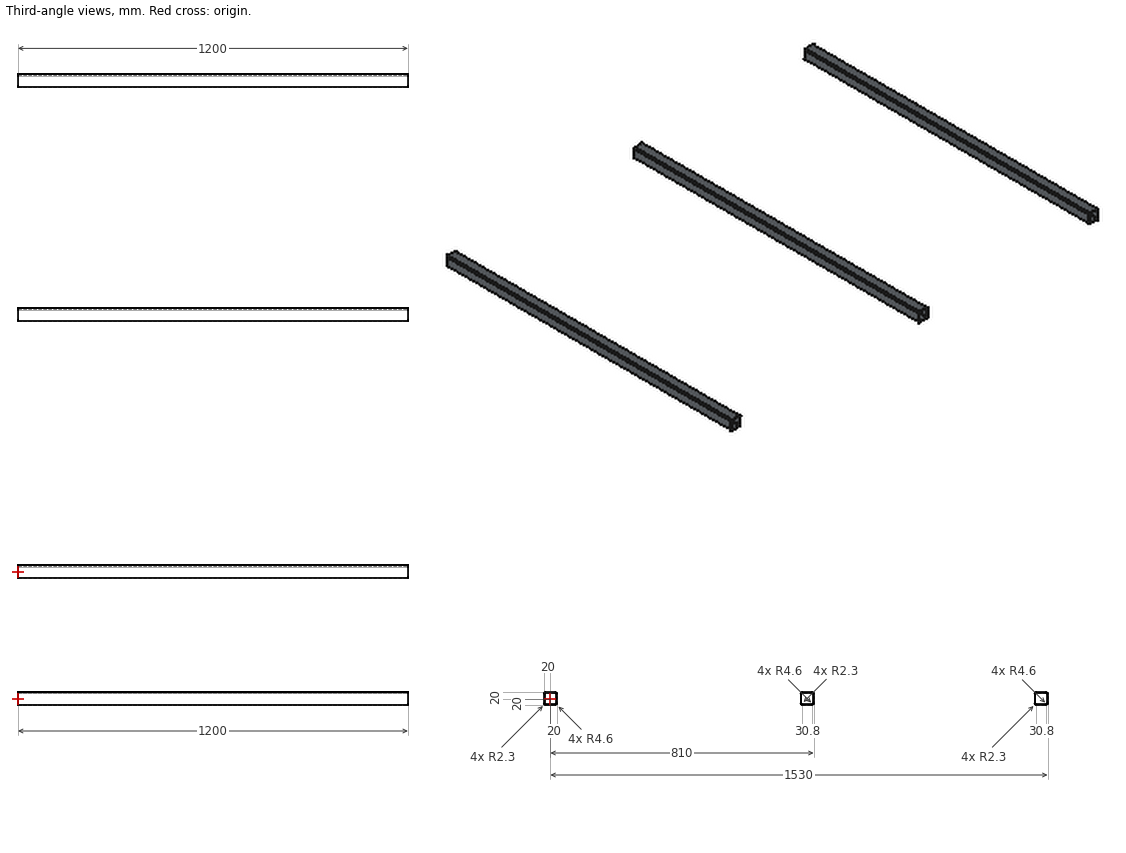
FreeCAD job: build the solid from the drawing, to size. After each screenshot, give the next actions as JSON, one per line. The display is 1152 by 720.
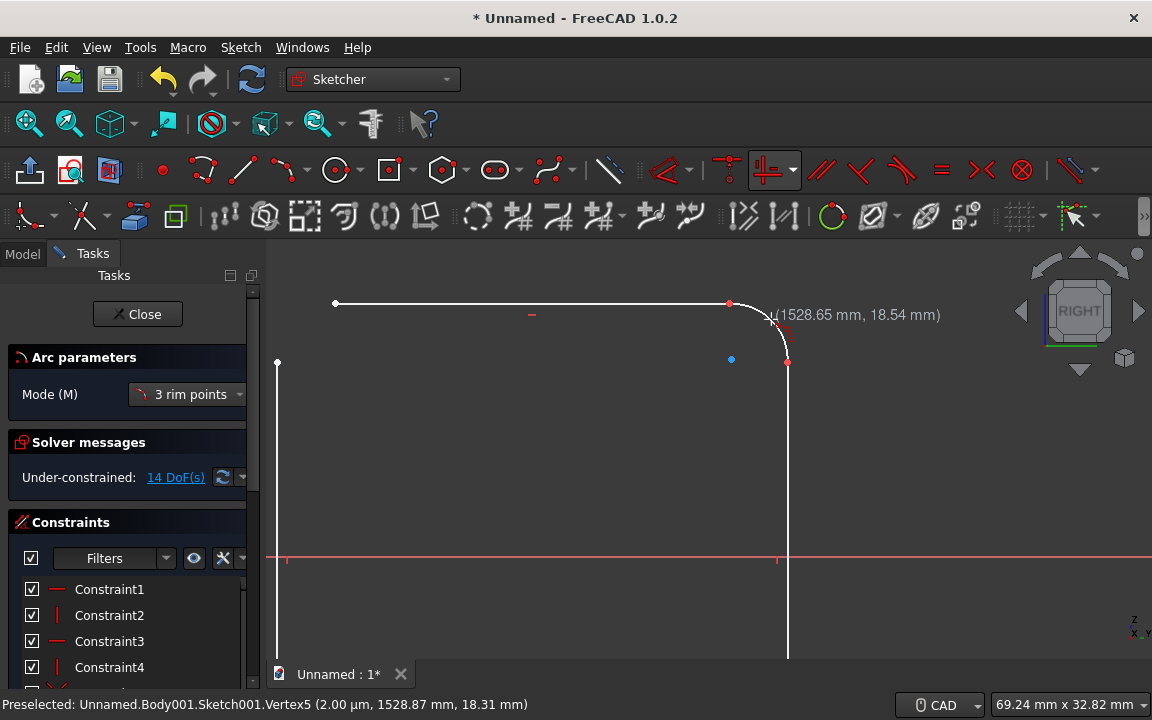
{"action": "left_click", "coordinate": [336, 304]}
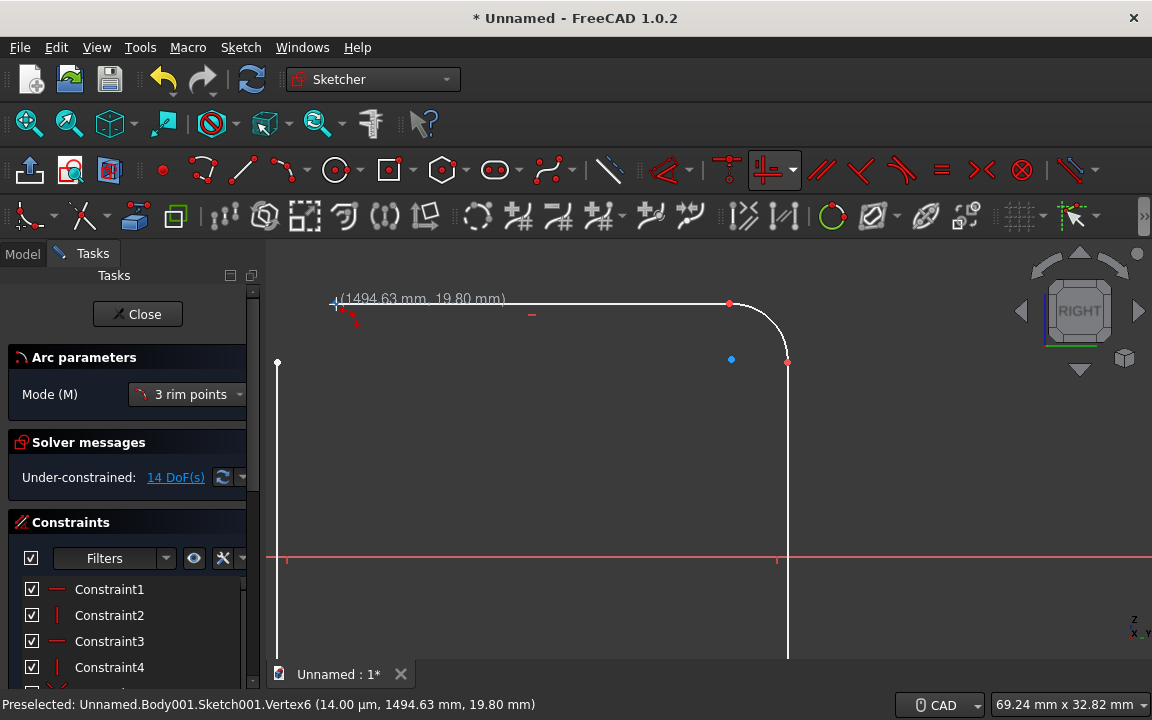
{"action": "scroll", "coordinate": [772, 317], "scroll_direction": "down", "scroll_amount": 3}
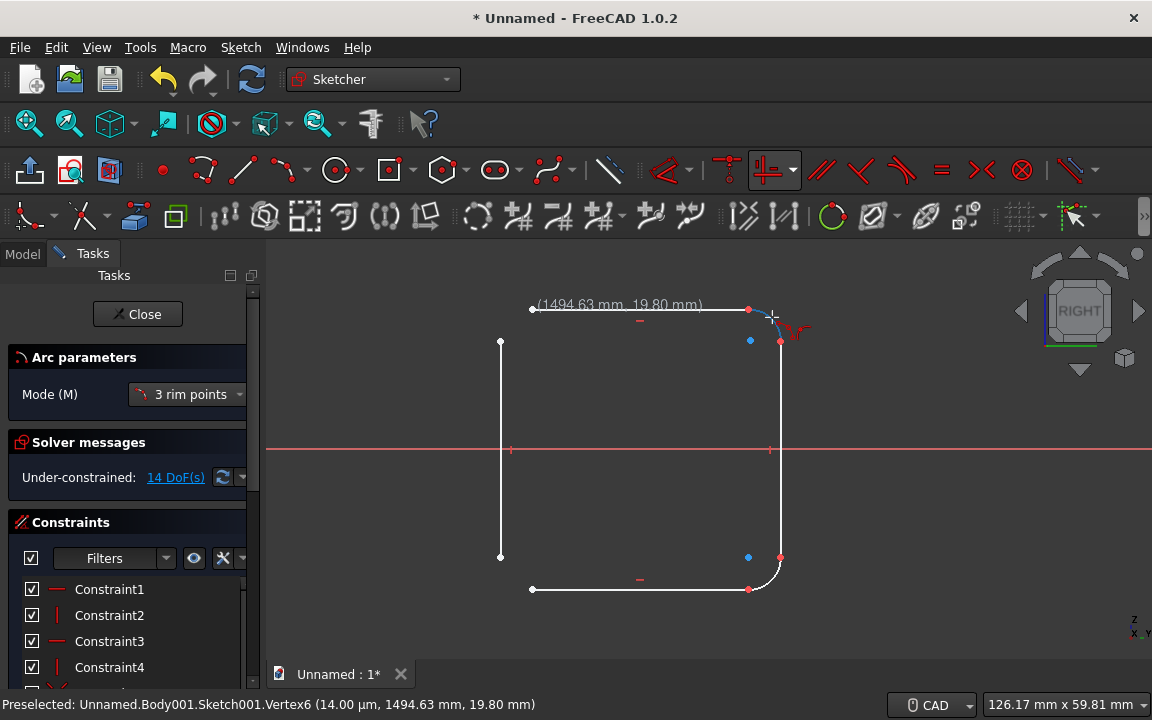
{"action": "left_click", "coordinate": [501, 342]}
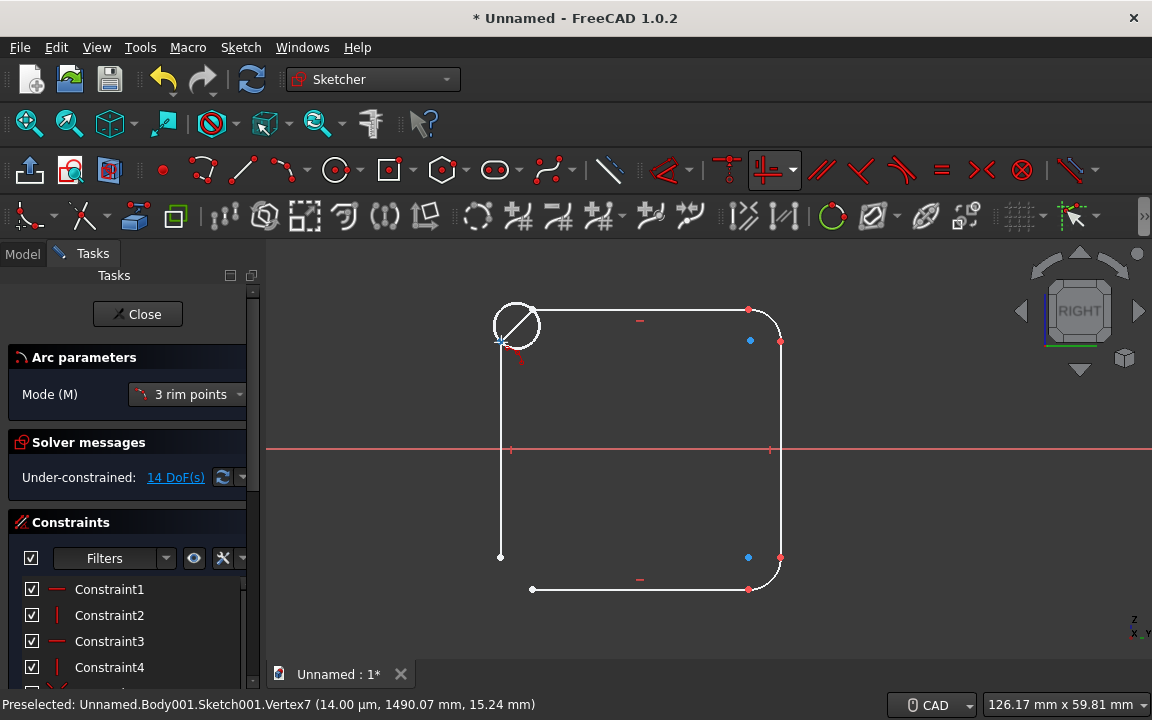
{"action": "scroll", "coordinate": [510, 318], "scroll_direction": "up", "scroll_amount": 3}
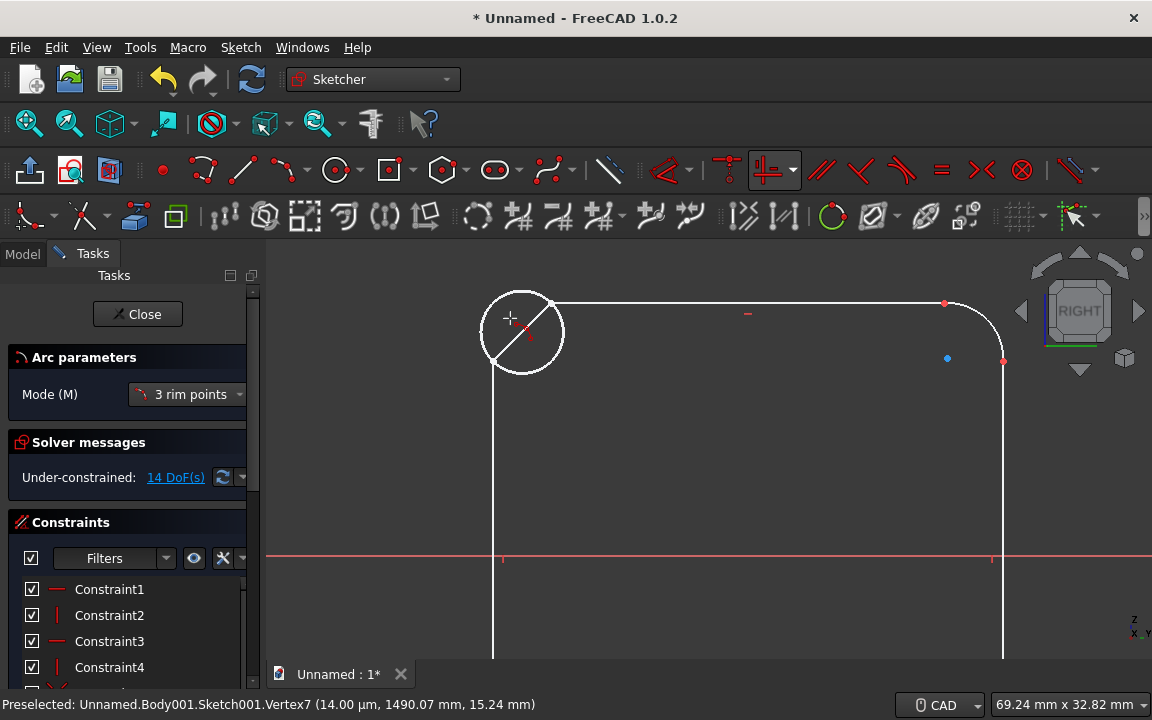
{"action": "left_click", "coordinate": [509, 318]}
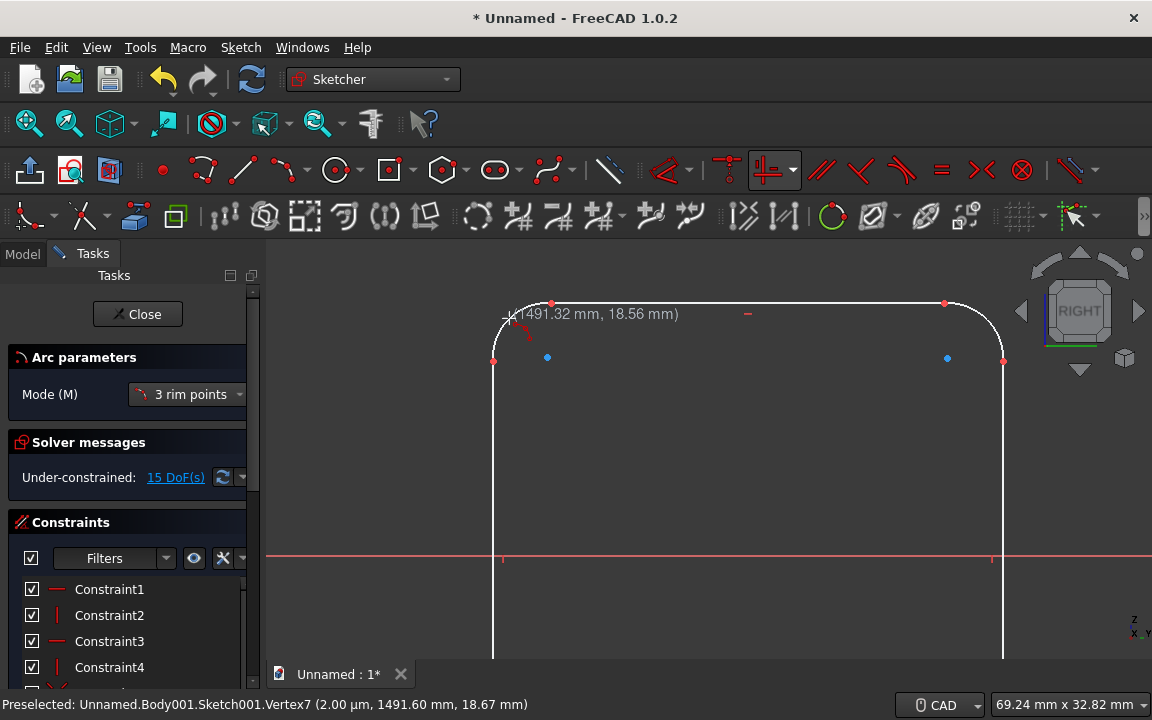
{"action": "scroll", "coordinate": [510, 318], "scroll_direction": "down", "scroll_amount": 3}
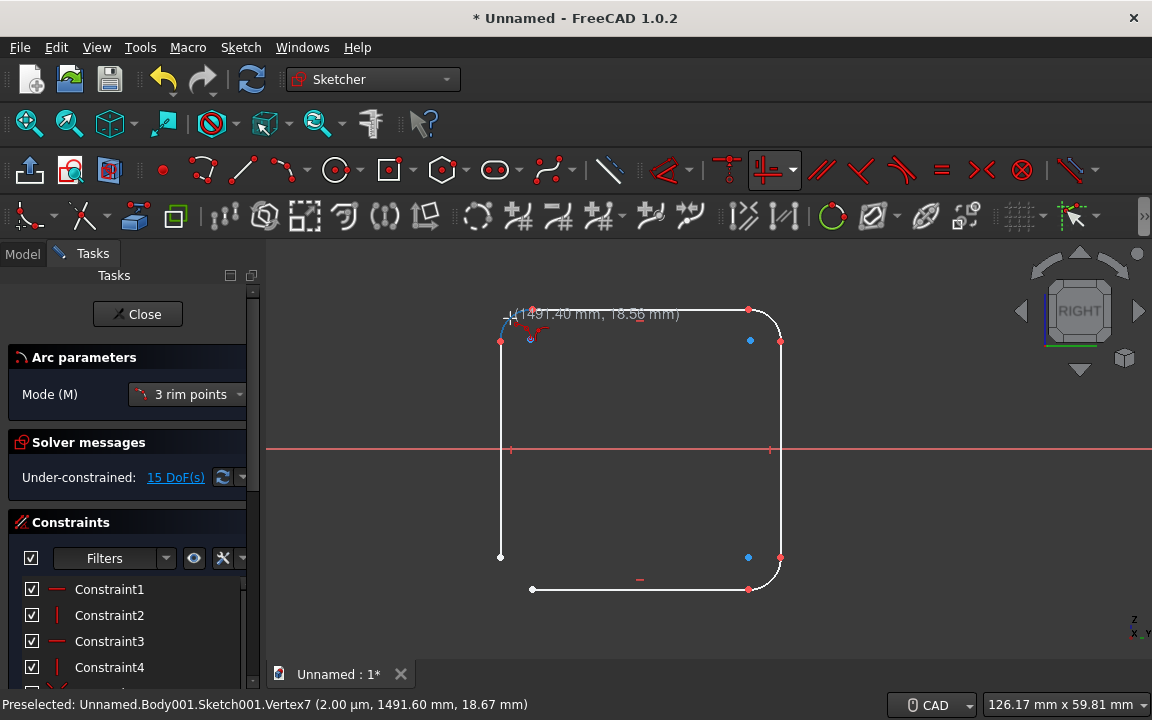
{"action": "left_click", "coordinate": [501, 558]}
{"action": "left_click", "coordinate": [533, 590]}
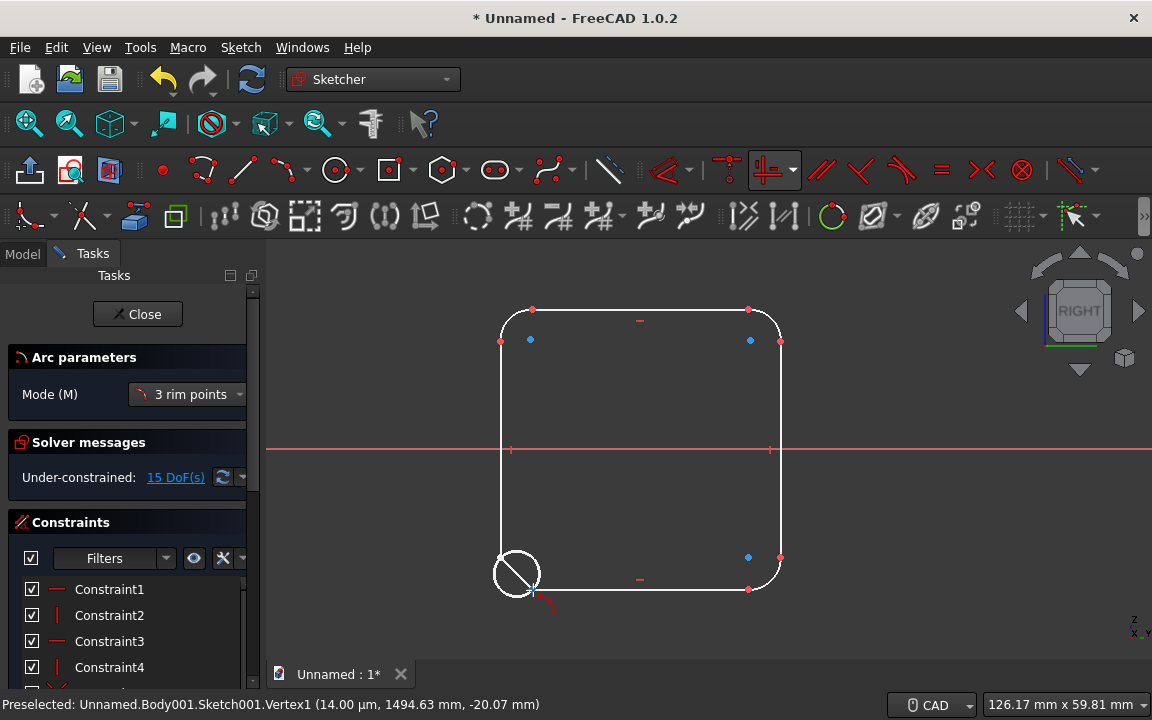
{"action": "scroll", "coordinate": [510, 580], "scroll_direction": "up", "scroll_amount": 3}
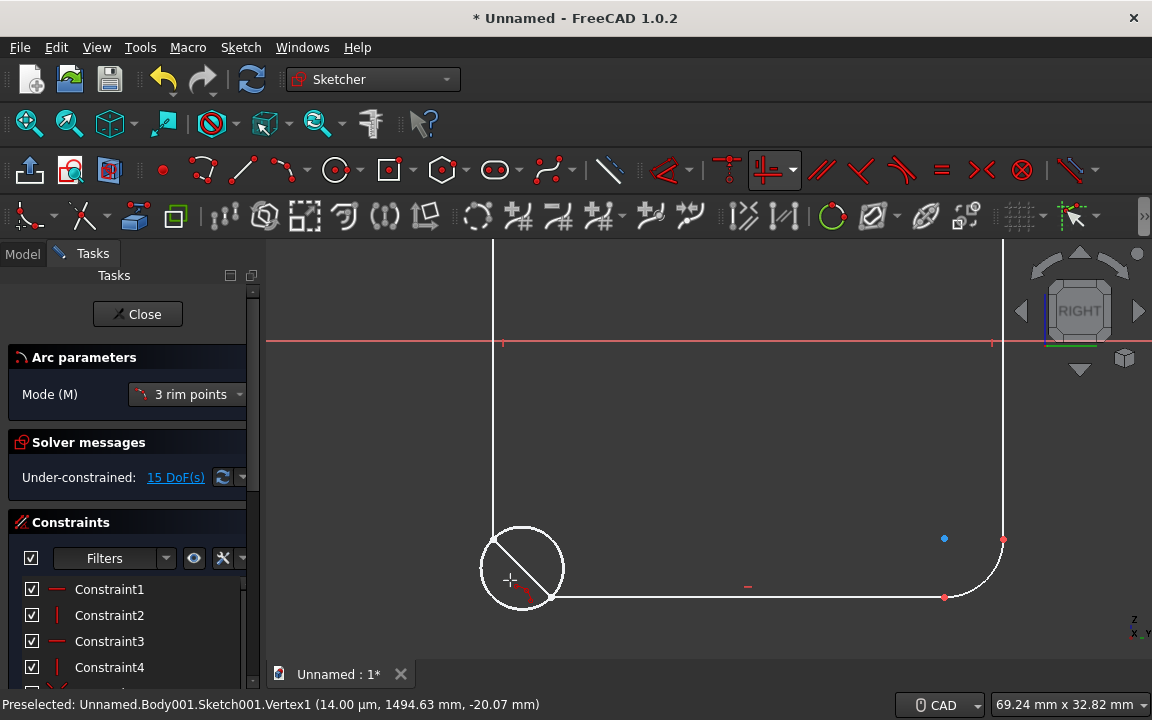
{"action": "left_click", "coordinate": [509, 579]}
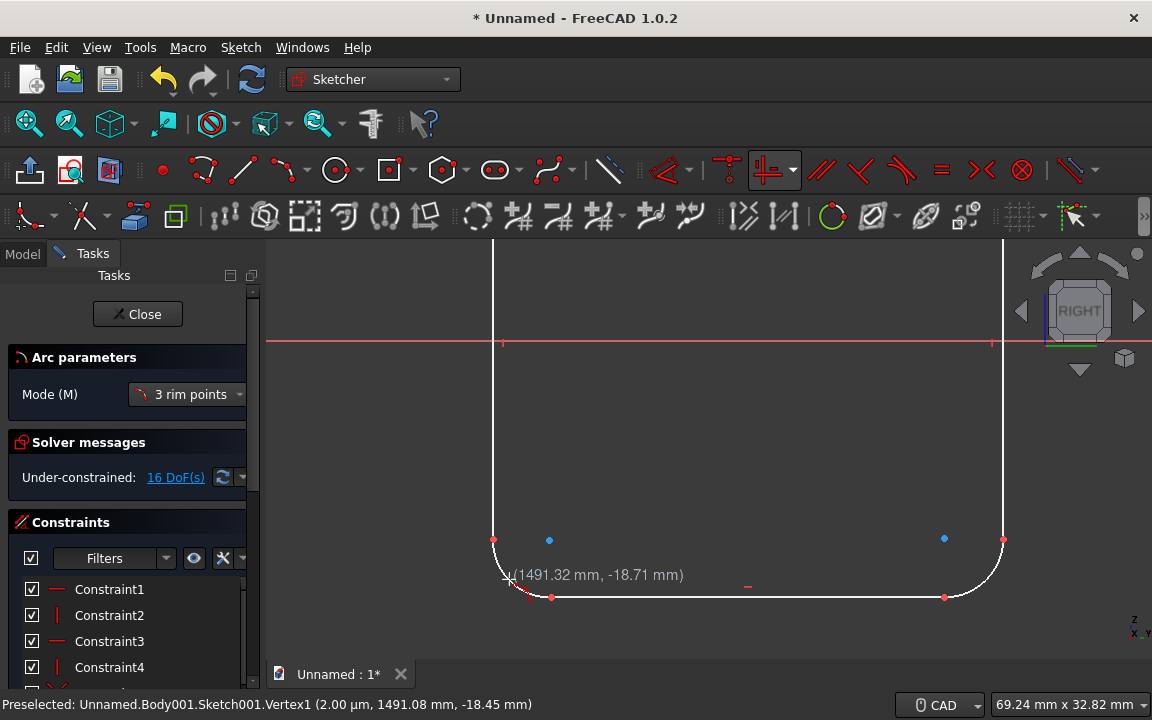
{"action": "left_click", "coordinate": [244, 170]}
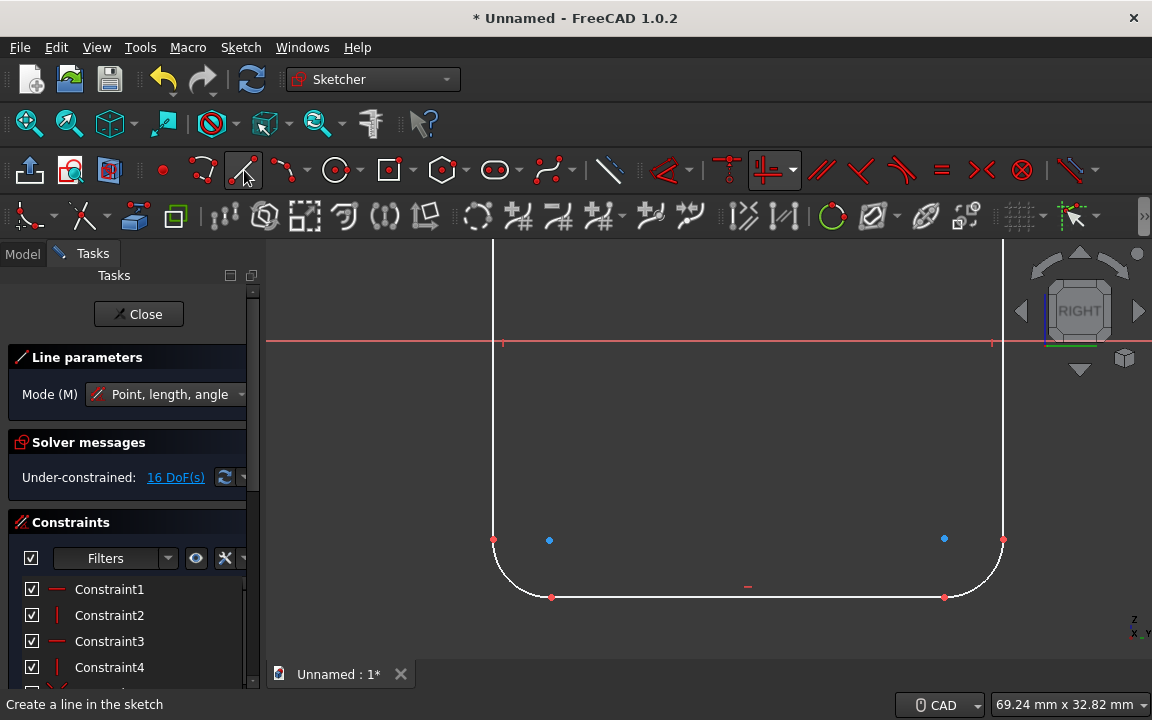
{"action": "left_click", "coordinate": [945, 567]}
{"action": "left_click", "coordinate": [551, 567]}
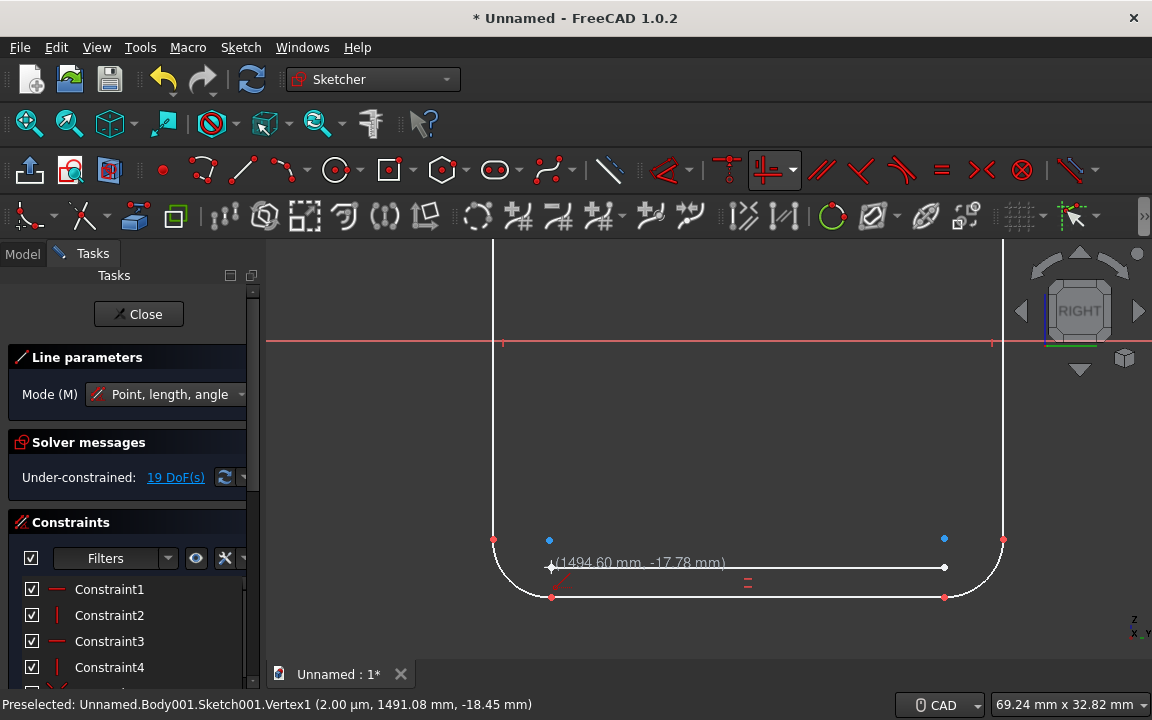
{"action": "left_click", "coordinate": [522, 538]}